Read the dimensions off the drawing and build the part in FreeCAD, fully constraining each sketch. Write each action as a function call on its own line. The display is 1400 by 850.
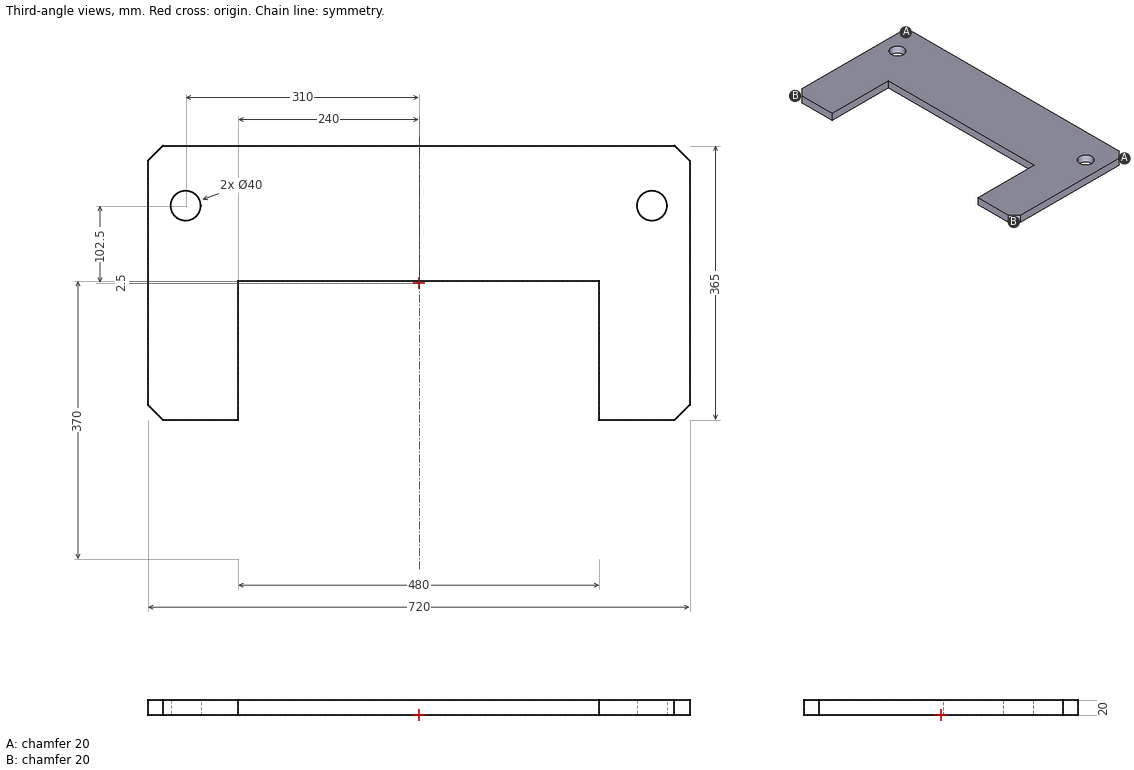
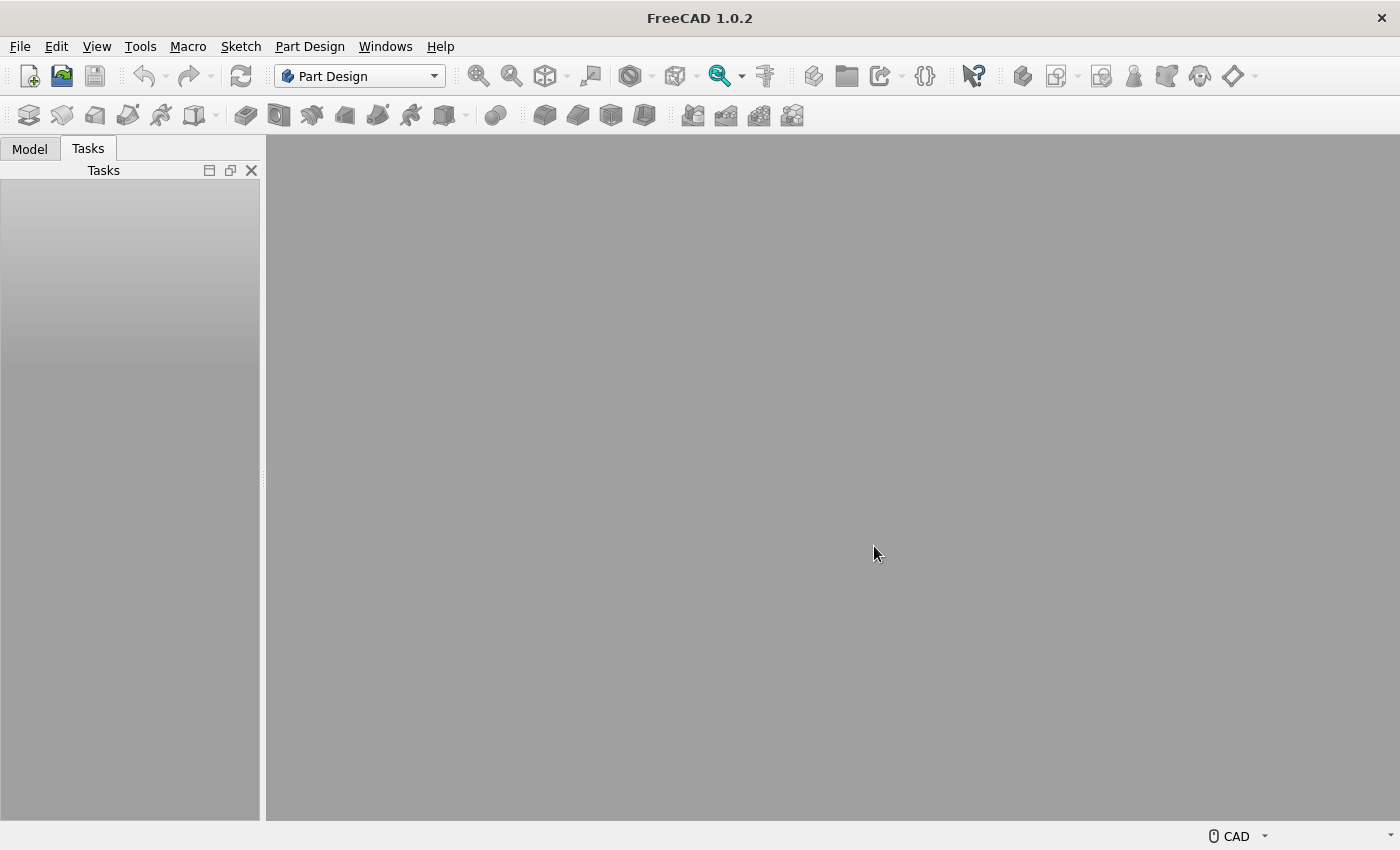
key(ctrl+n)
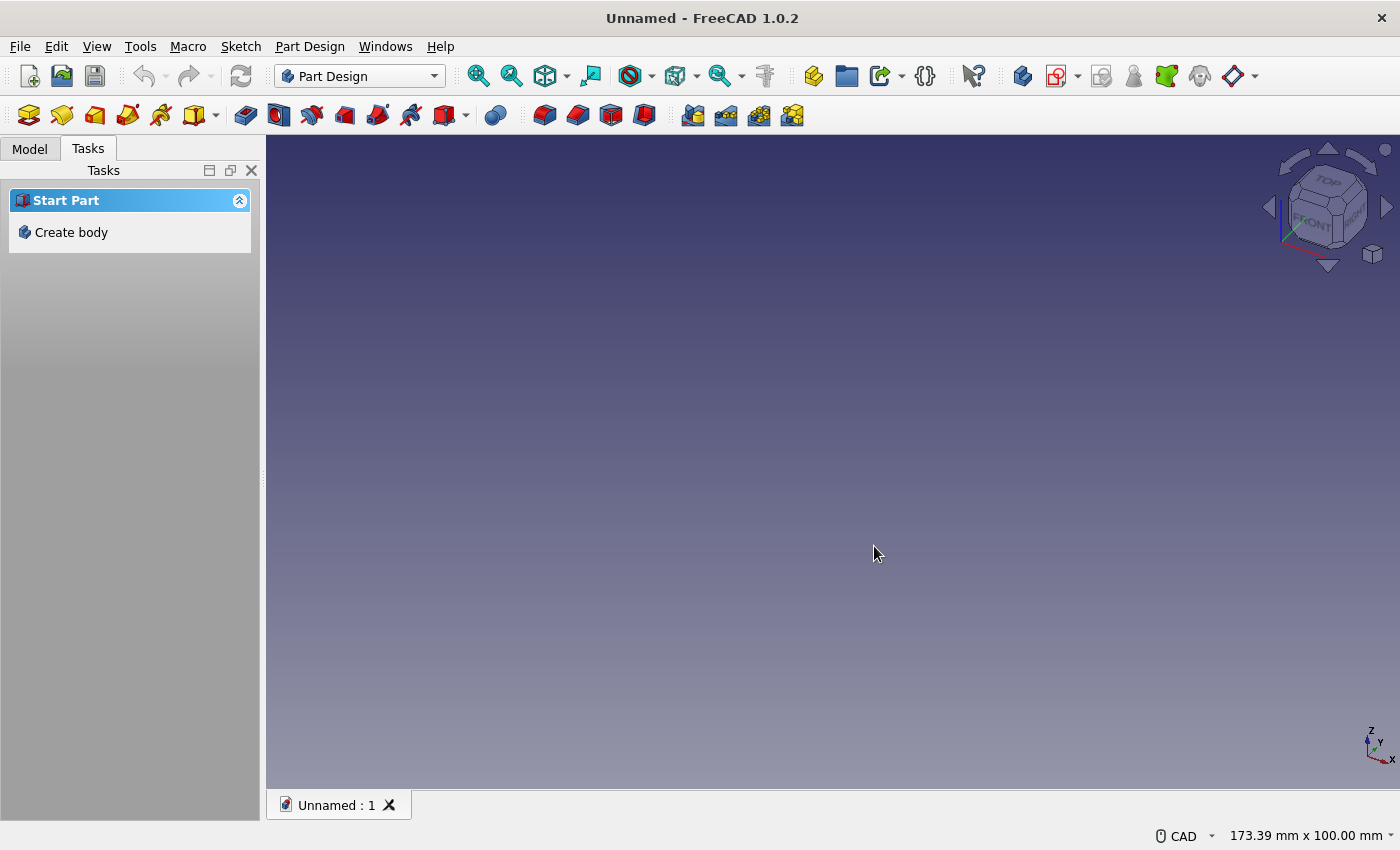
click(1056, 76)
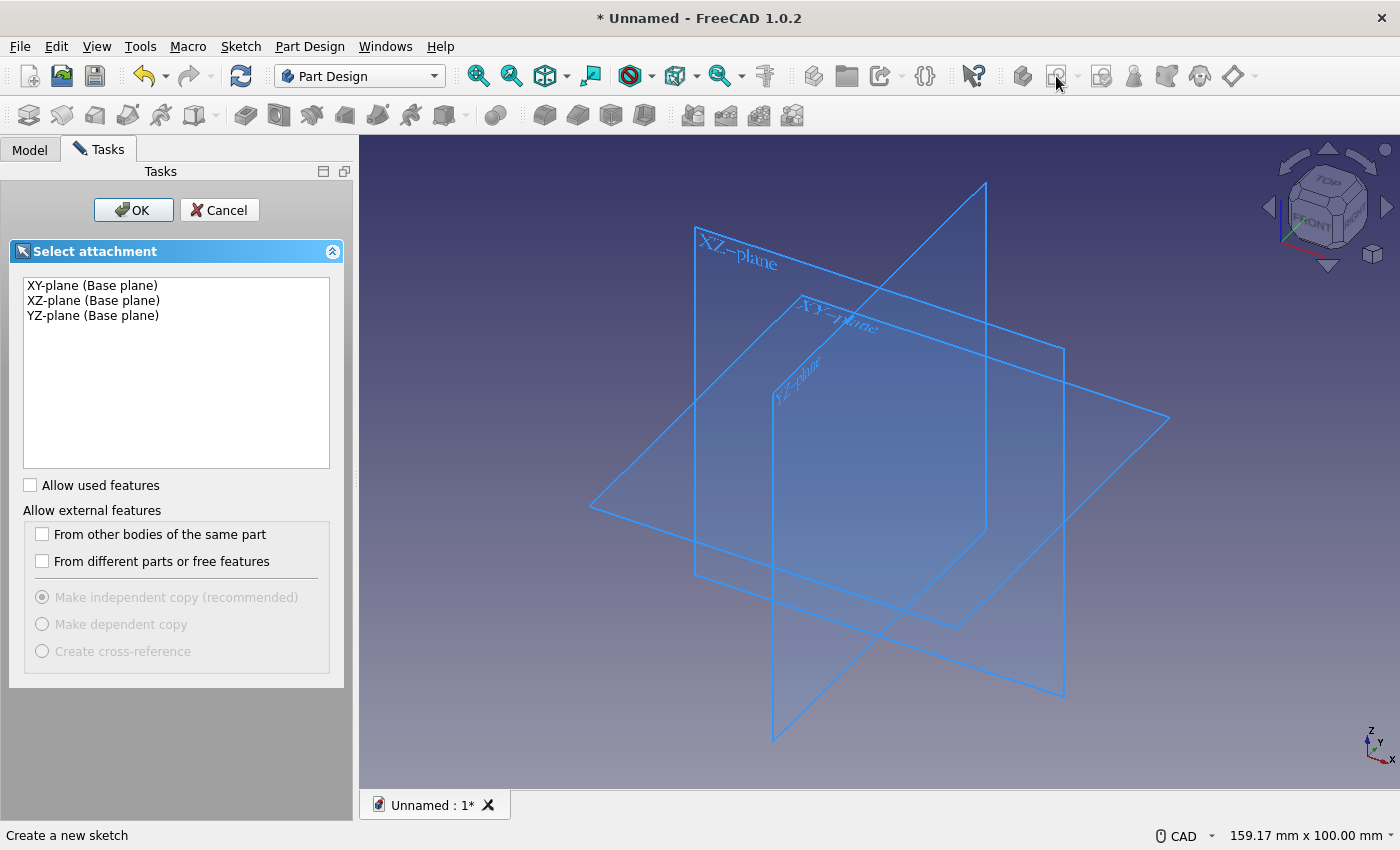
click(84, 286)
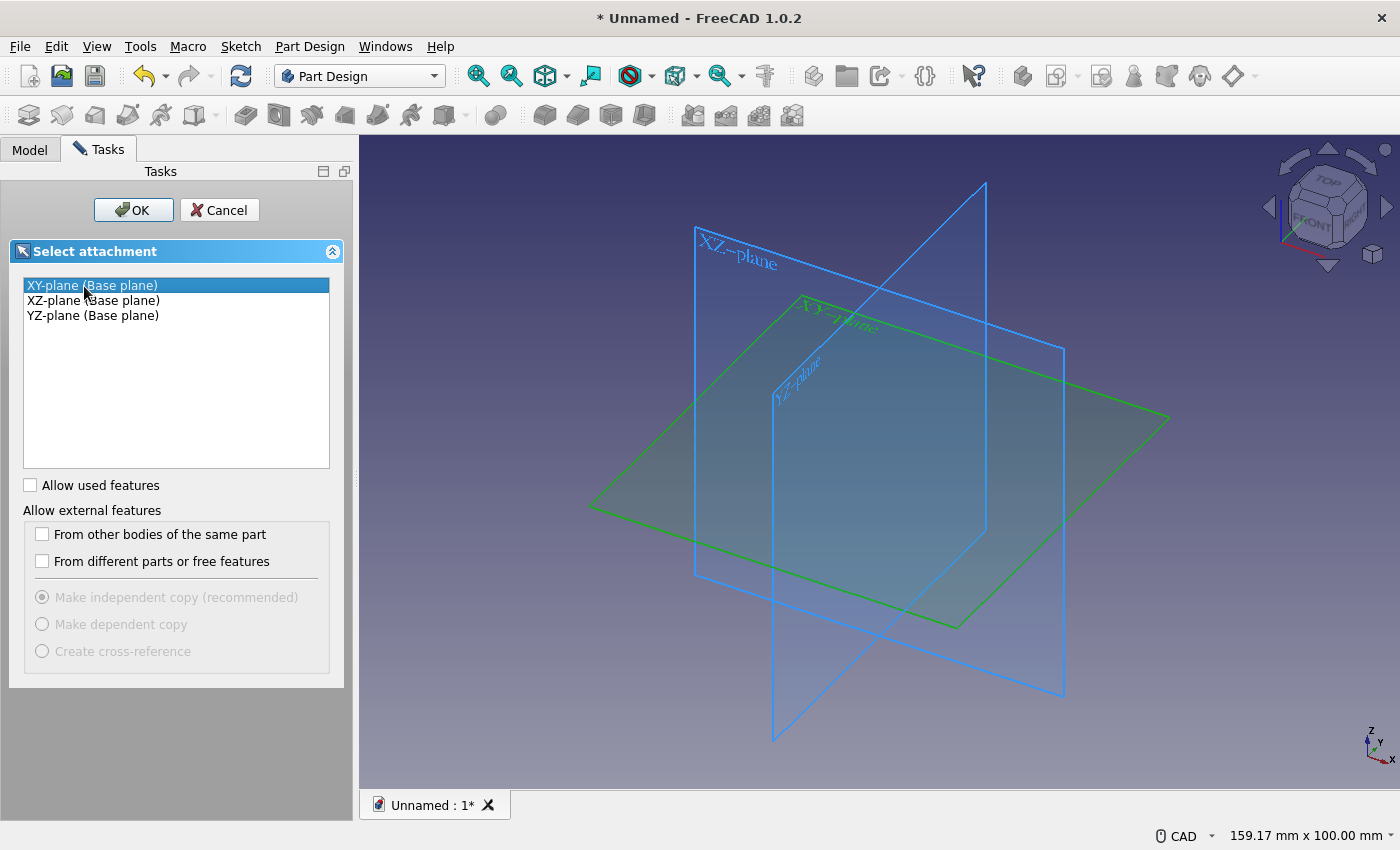
click(134, 210)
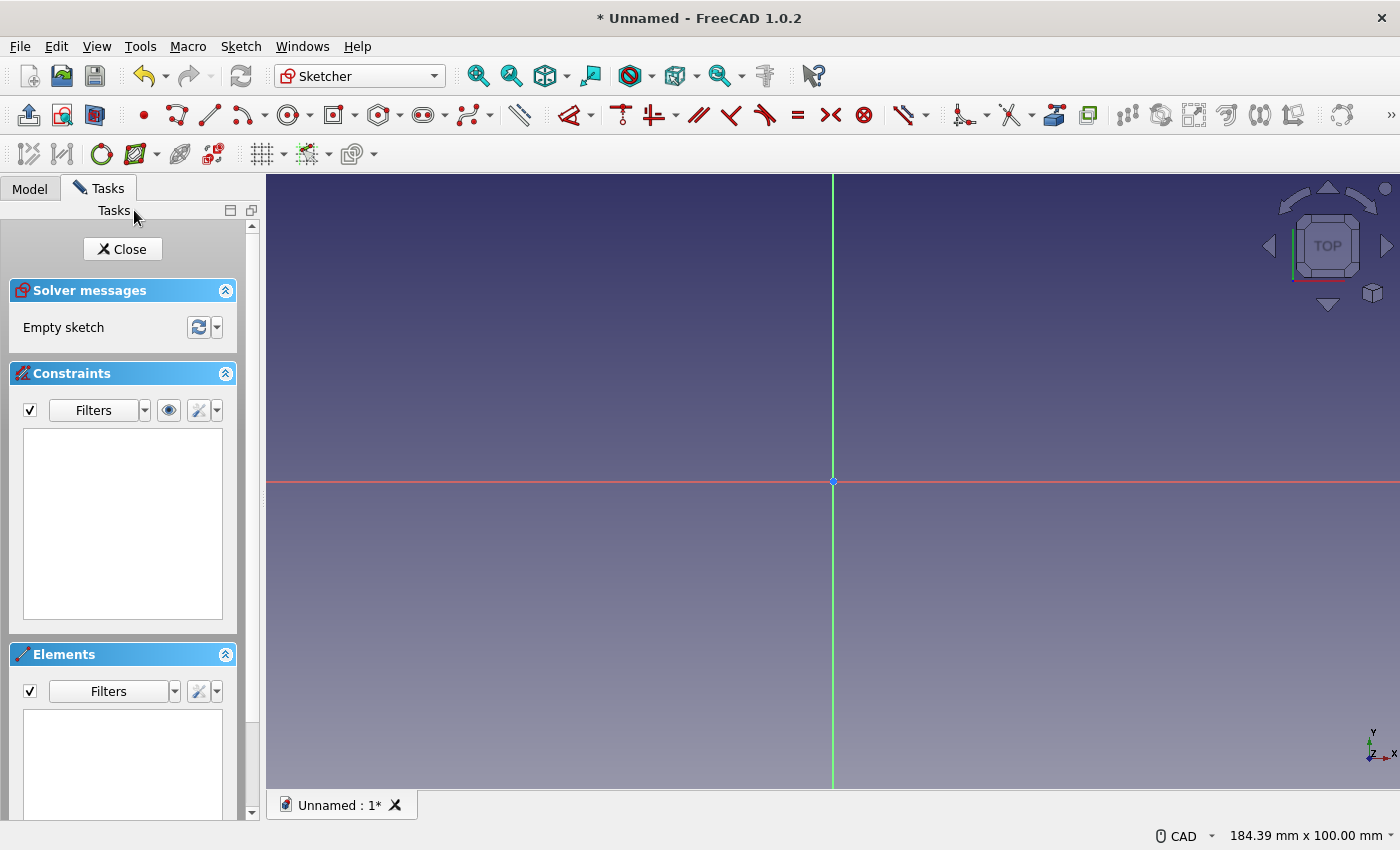
scroll(751, 482, down, 9)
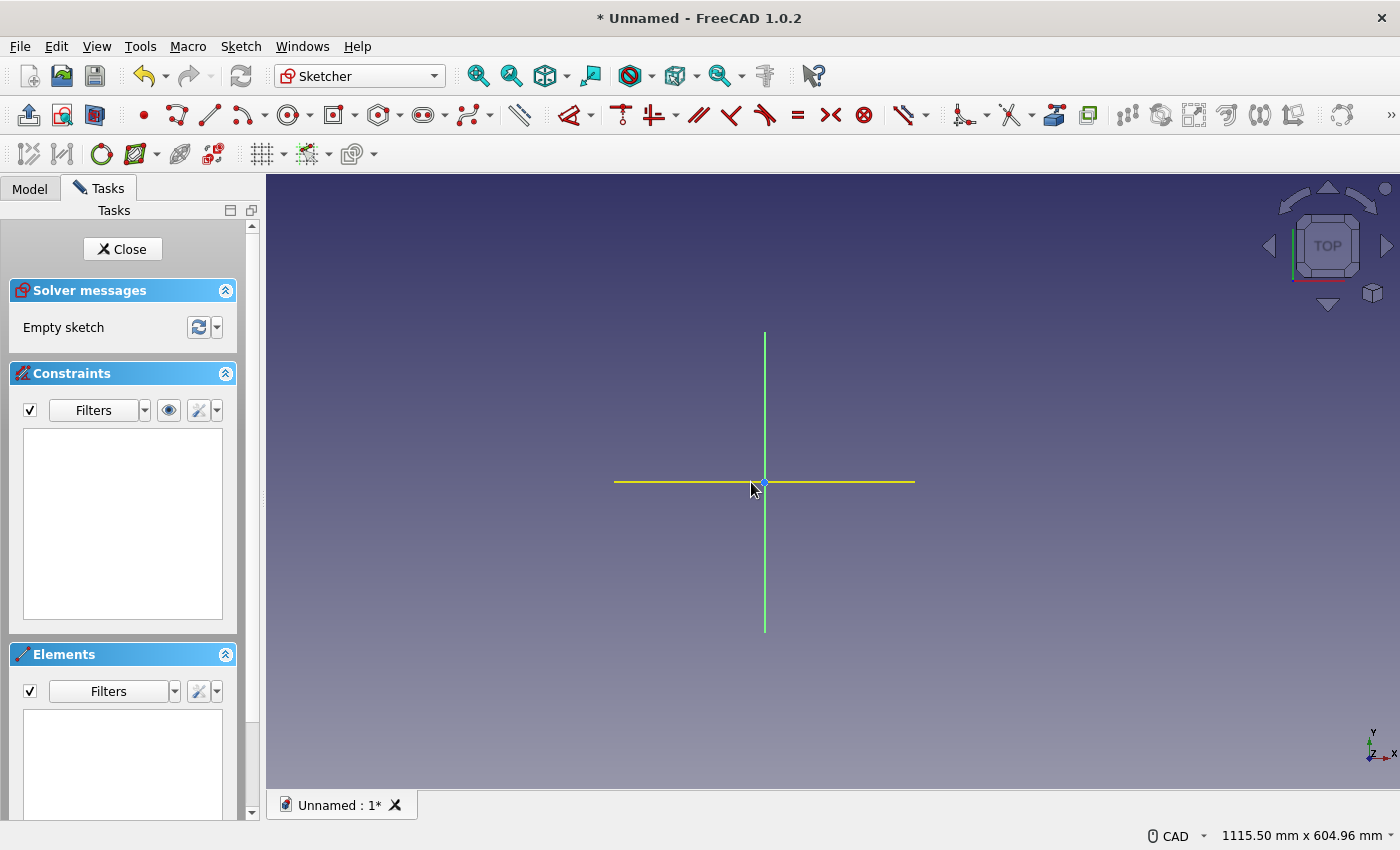
key(g)
key(v)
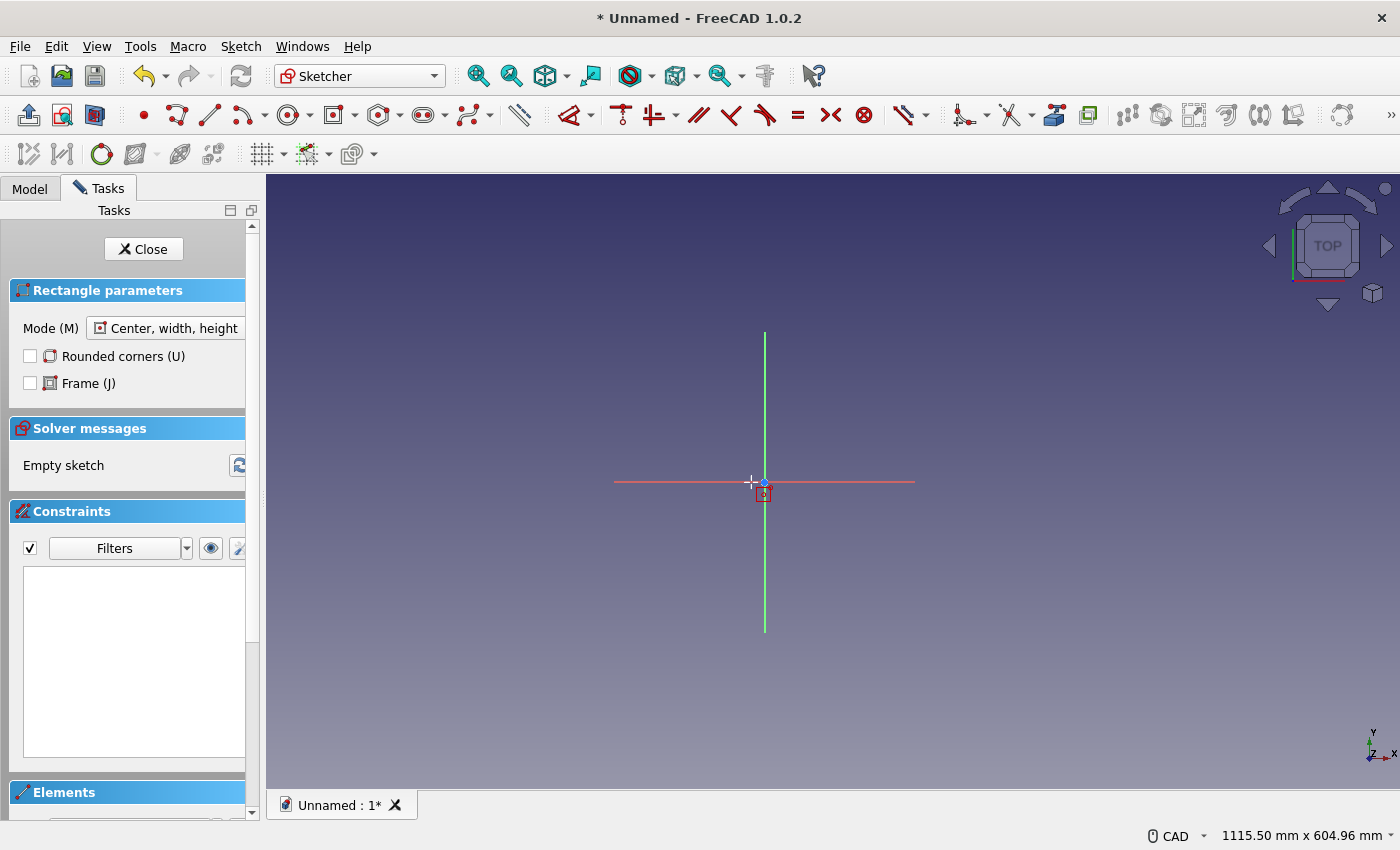
click(765, 482)
click(1131, 297)
key(Escape)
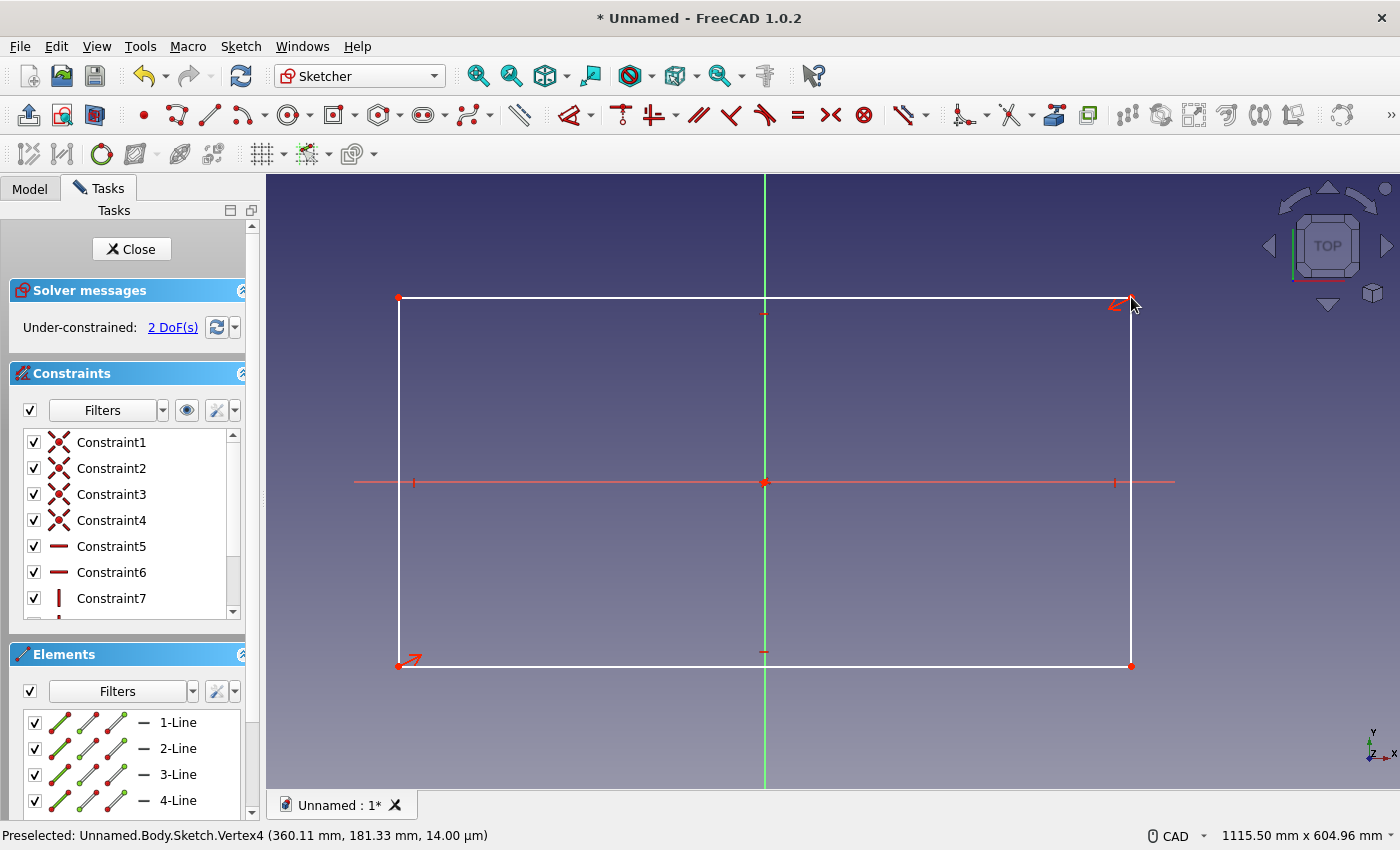
click(618, 667)